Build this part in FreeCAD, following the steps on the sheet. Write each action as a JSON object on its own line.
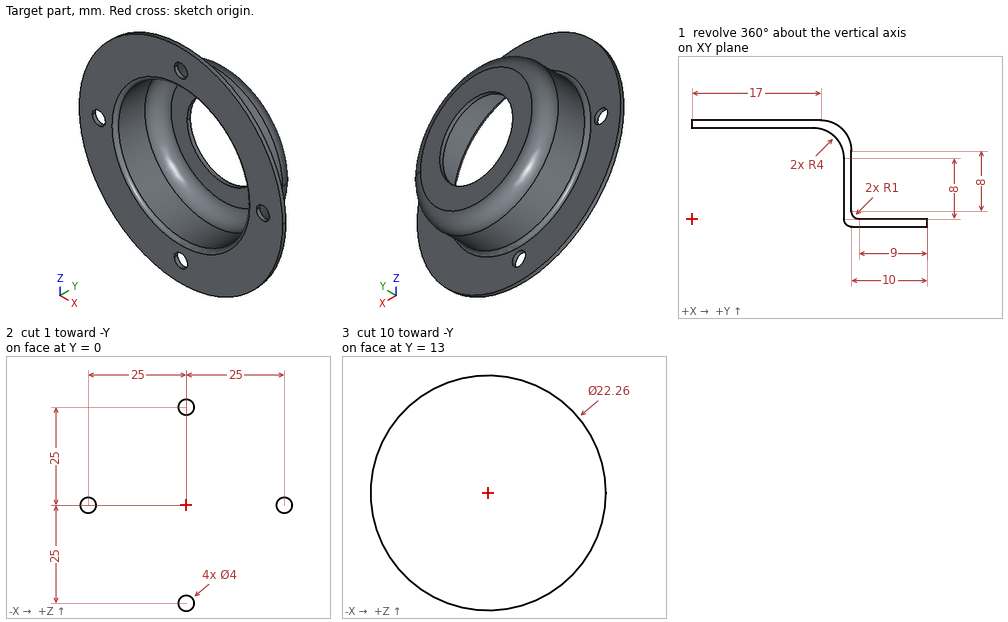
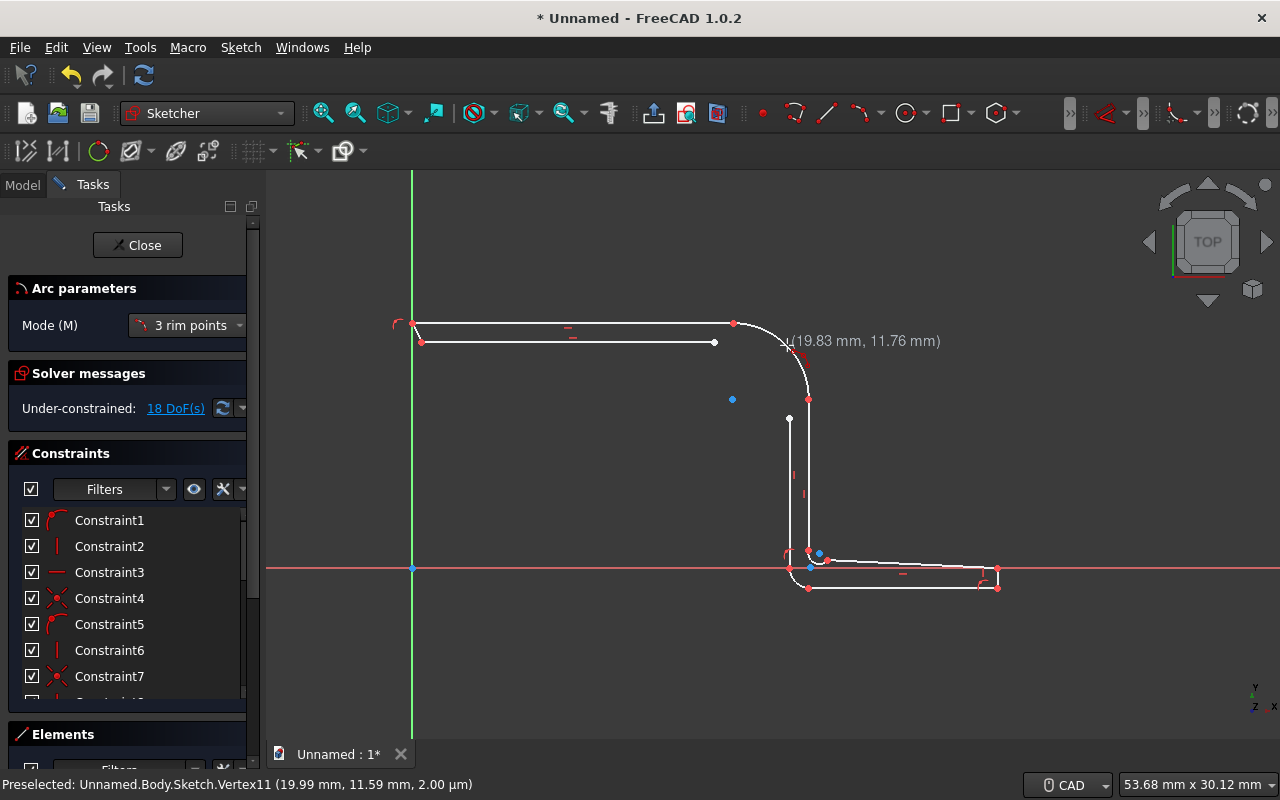
{"action": "left_click", "coordinate": [715, 342]}
{"action": "left_click", "coordinate": [790, 418]}
{"action": "left_click", "coordinate": [768, 364]}
{"action": "key", "text": "Escape"}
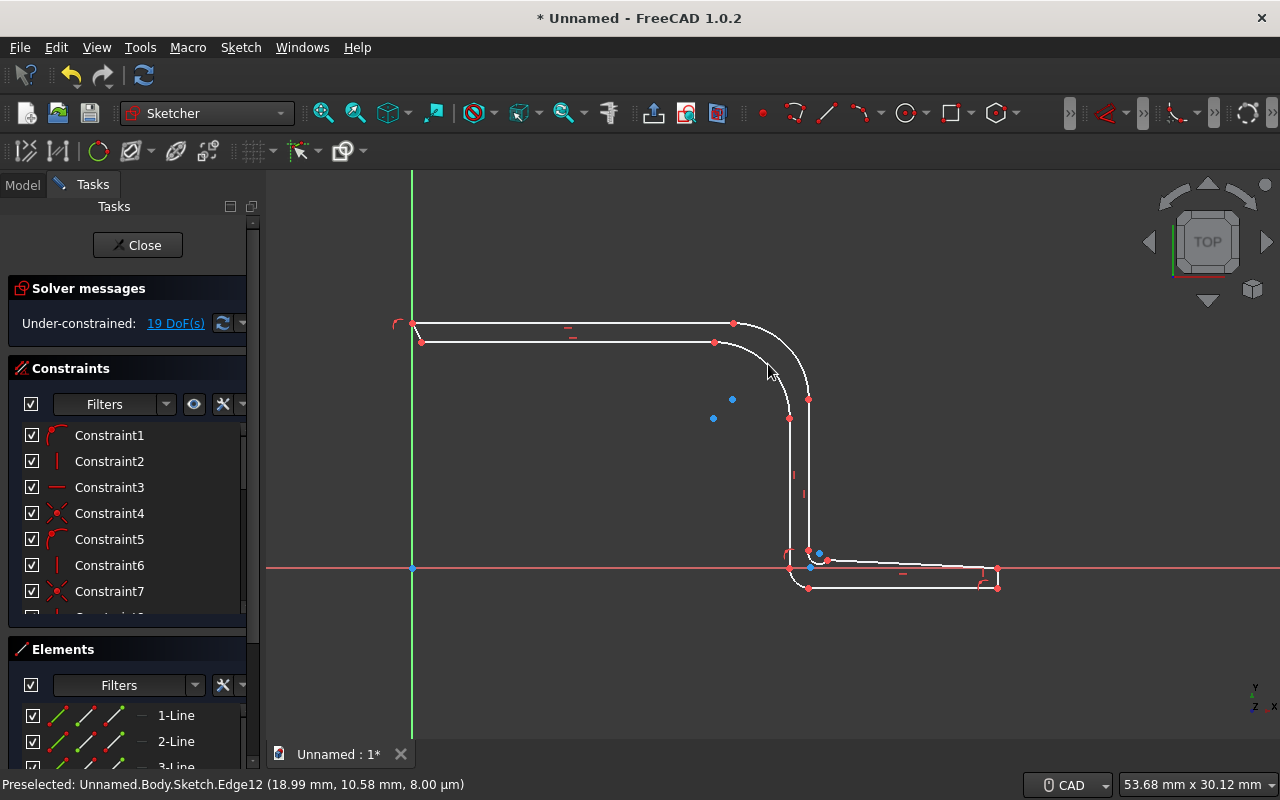
{"action": "left_click", "coordinate": [790, 463]}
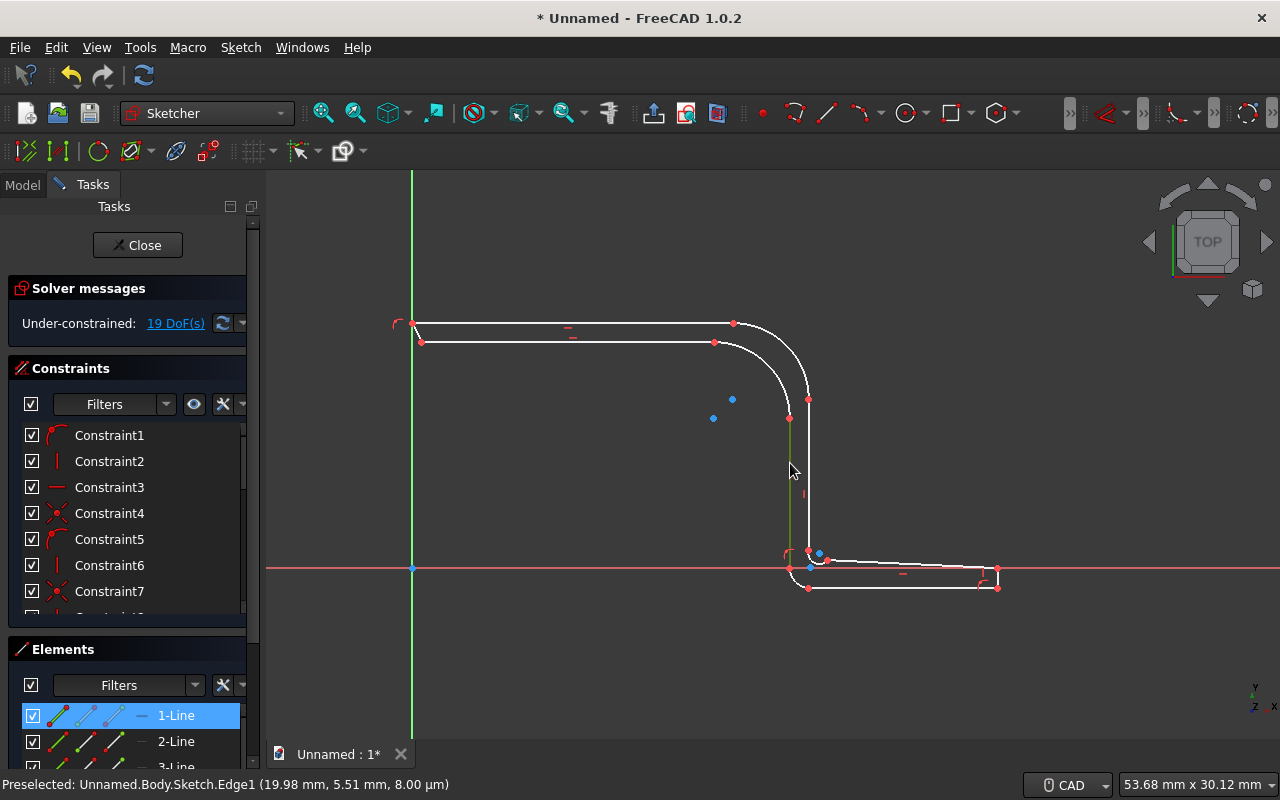
{"action": "left_click", "coordinate": [795, 582]}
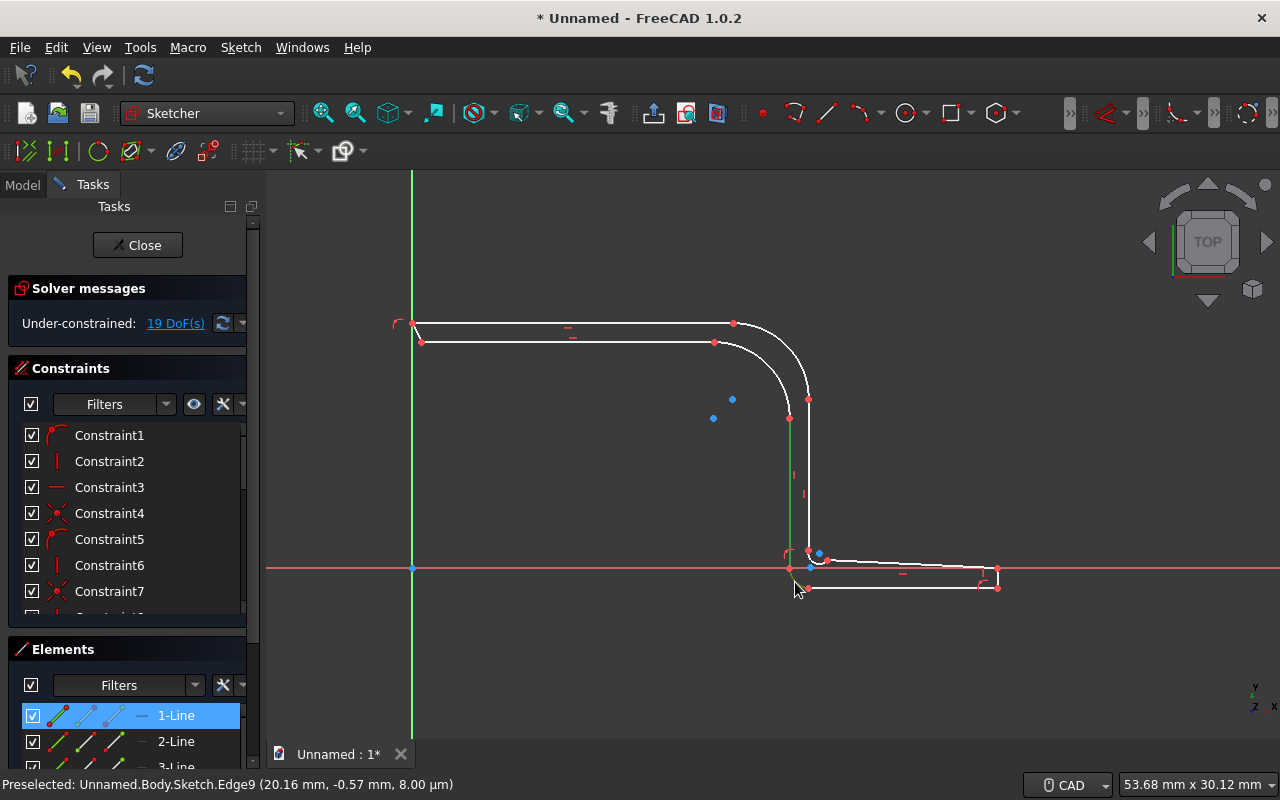
{"action": "key", "text": "t"}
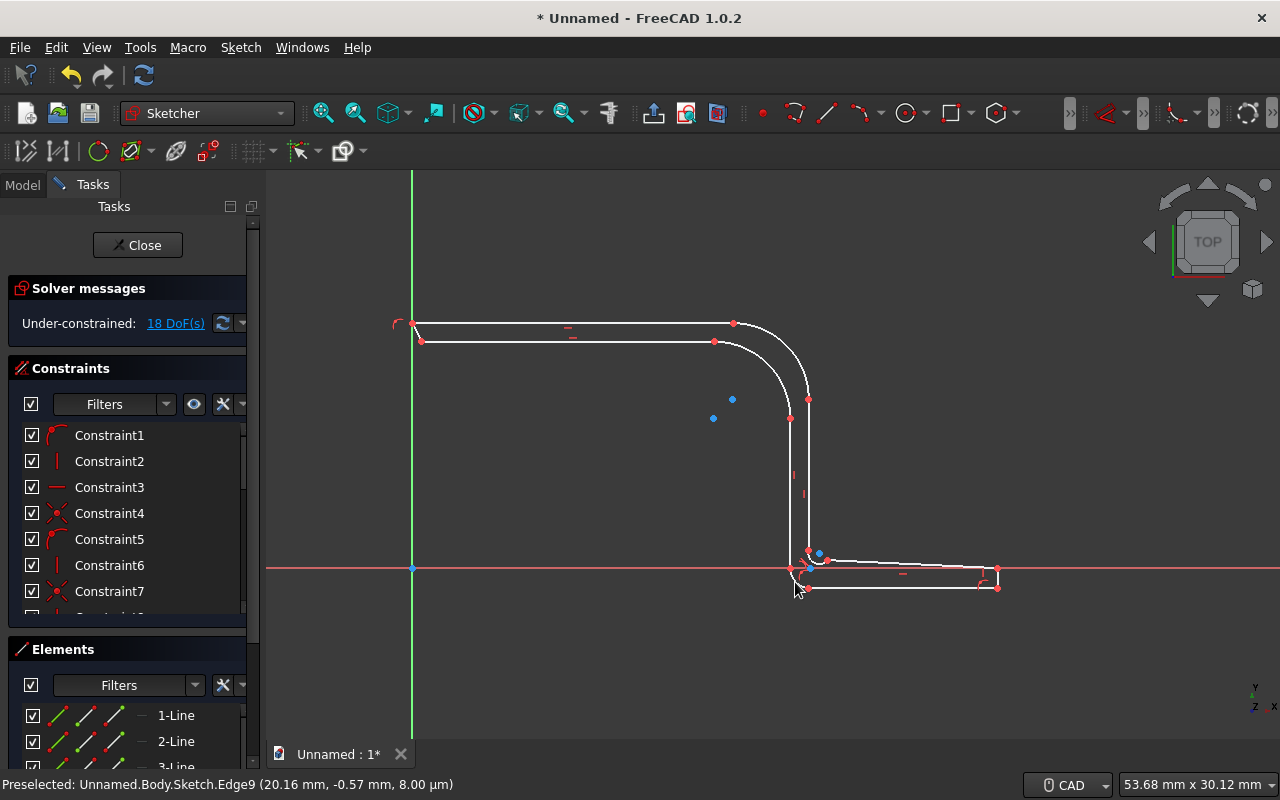
{"action": "left_click", "coordinate": [790, 463]}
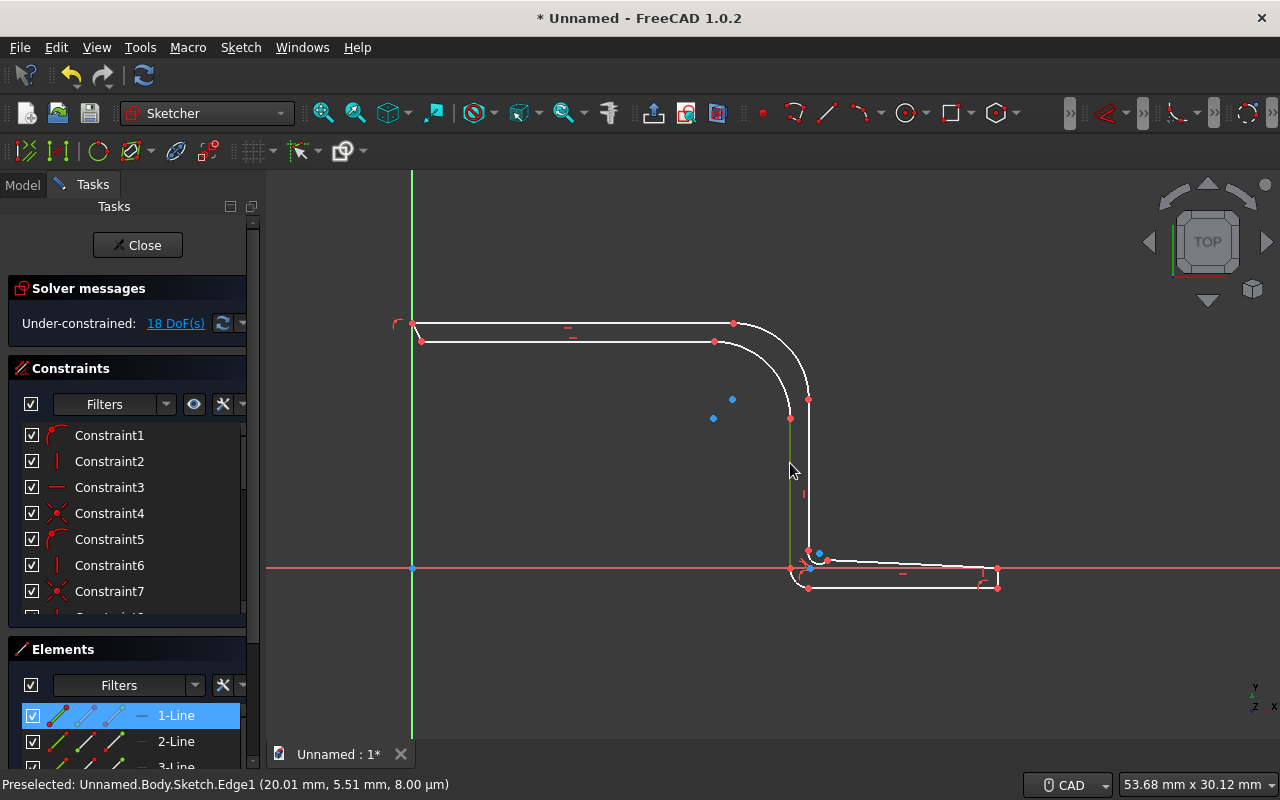
{"action": "left_click", "coordinate": [782, 384]}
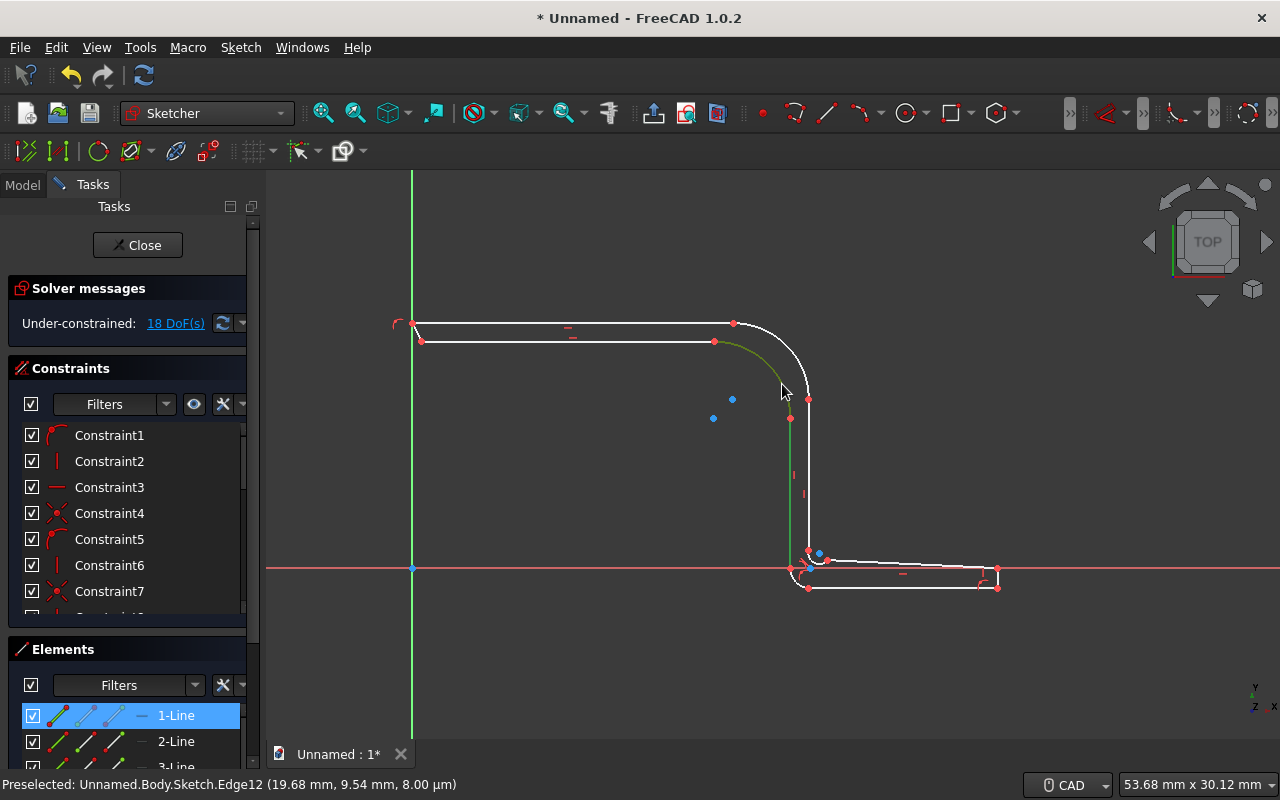
{"action": "key", "text": "t"}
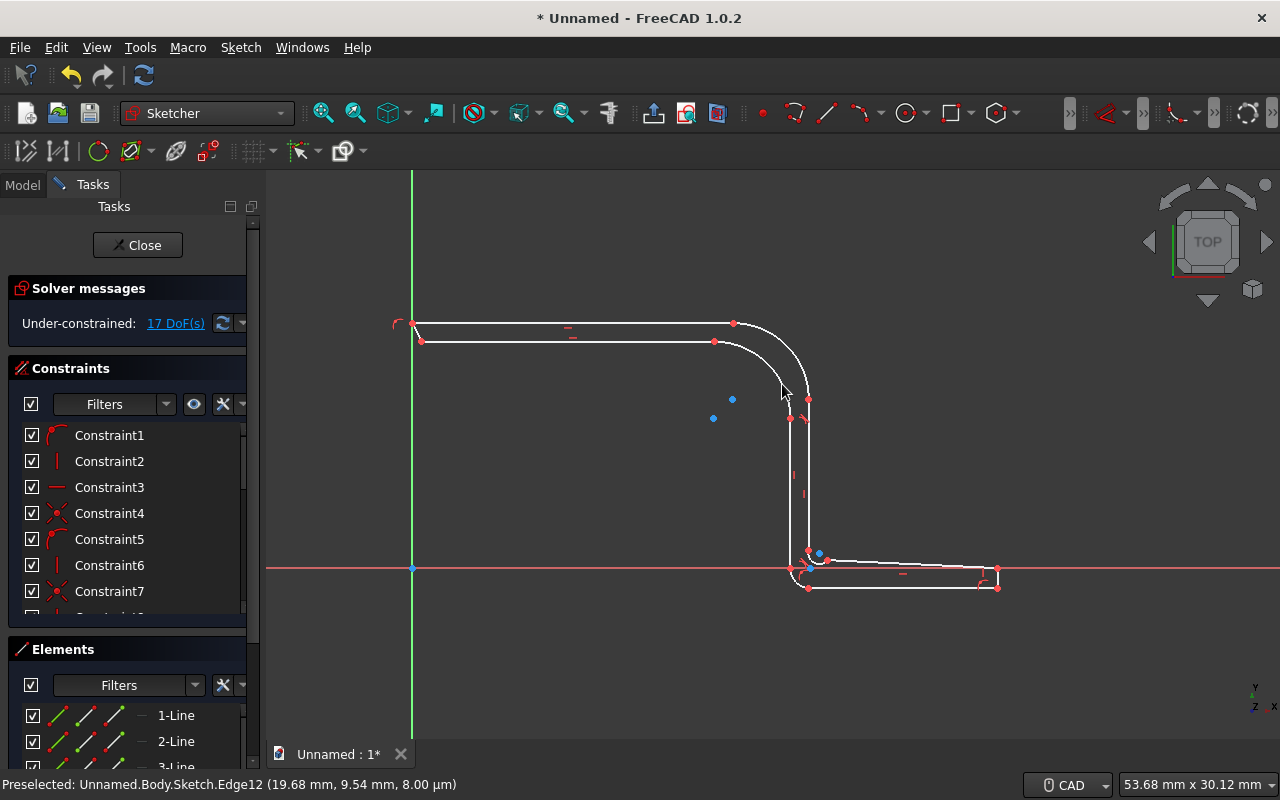
{"action": "left_click", "coordinate": [865, 588]}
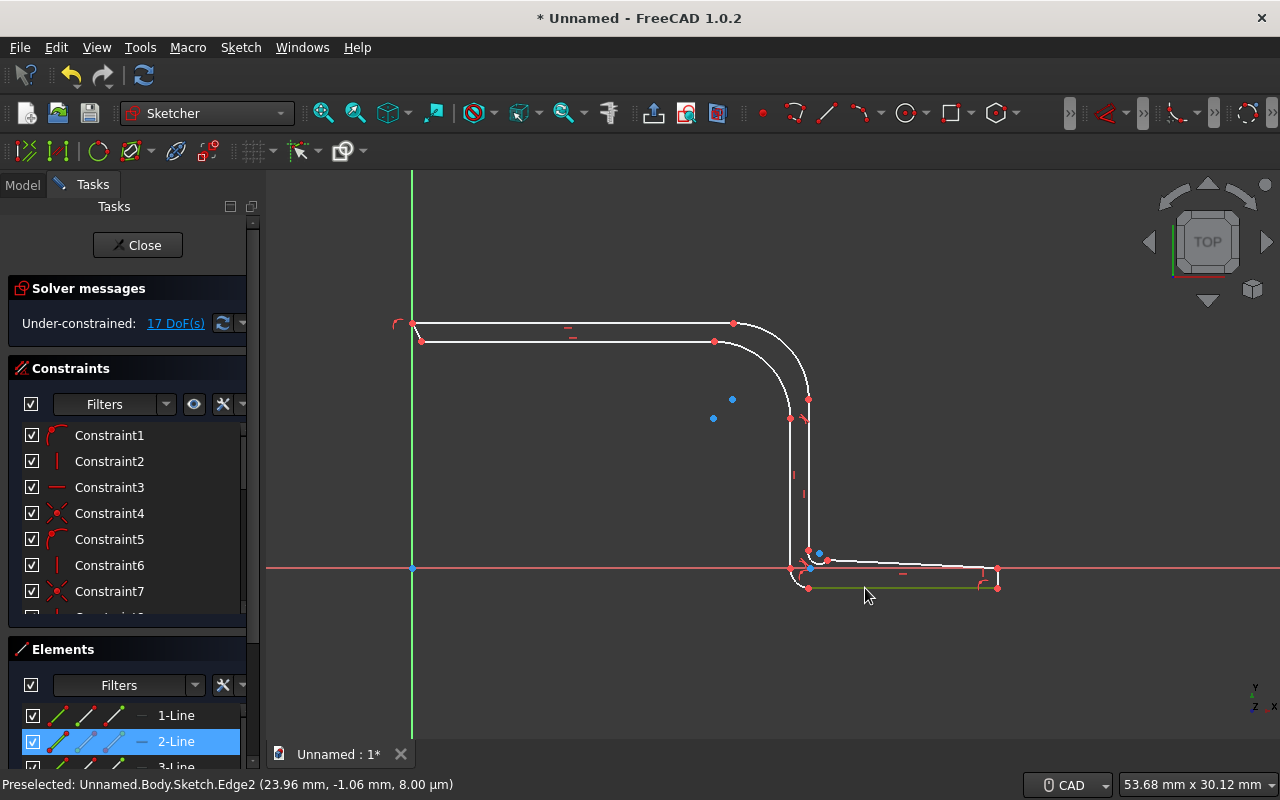
{"action": "left_click", "coordinate": [796, 582]}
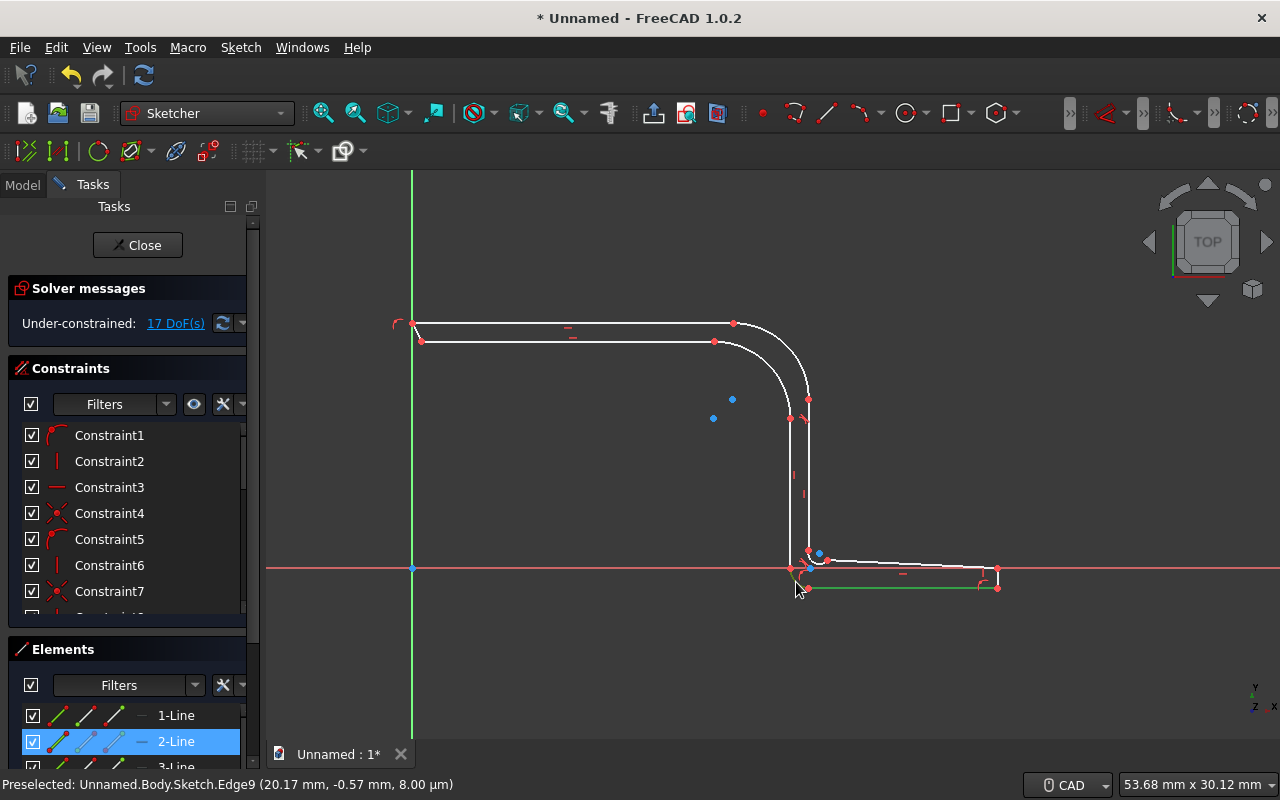
{"action": "key", "text": "t"}